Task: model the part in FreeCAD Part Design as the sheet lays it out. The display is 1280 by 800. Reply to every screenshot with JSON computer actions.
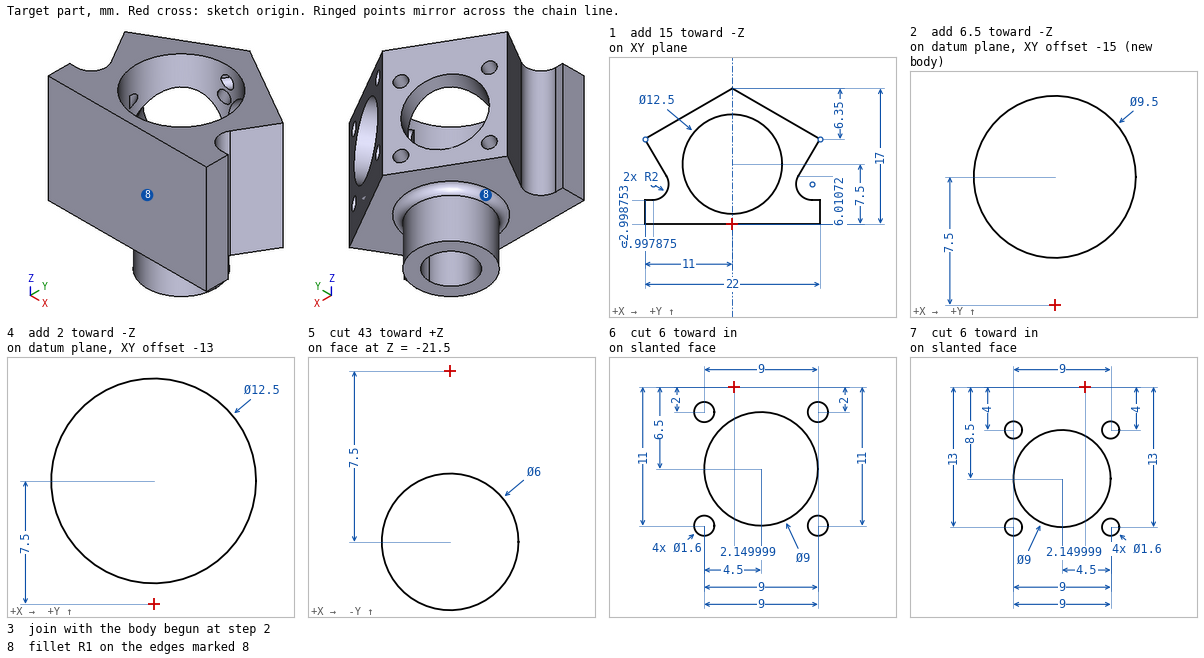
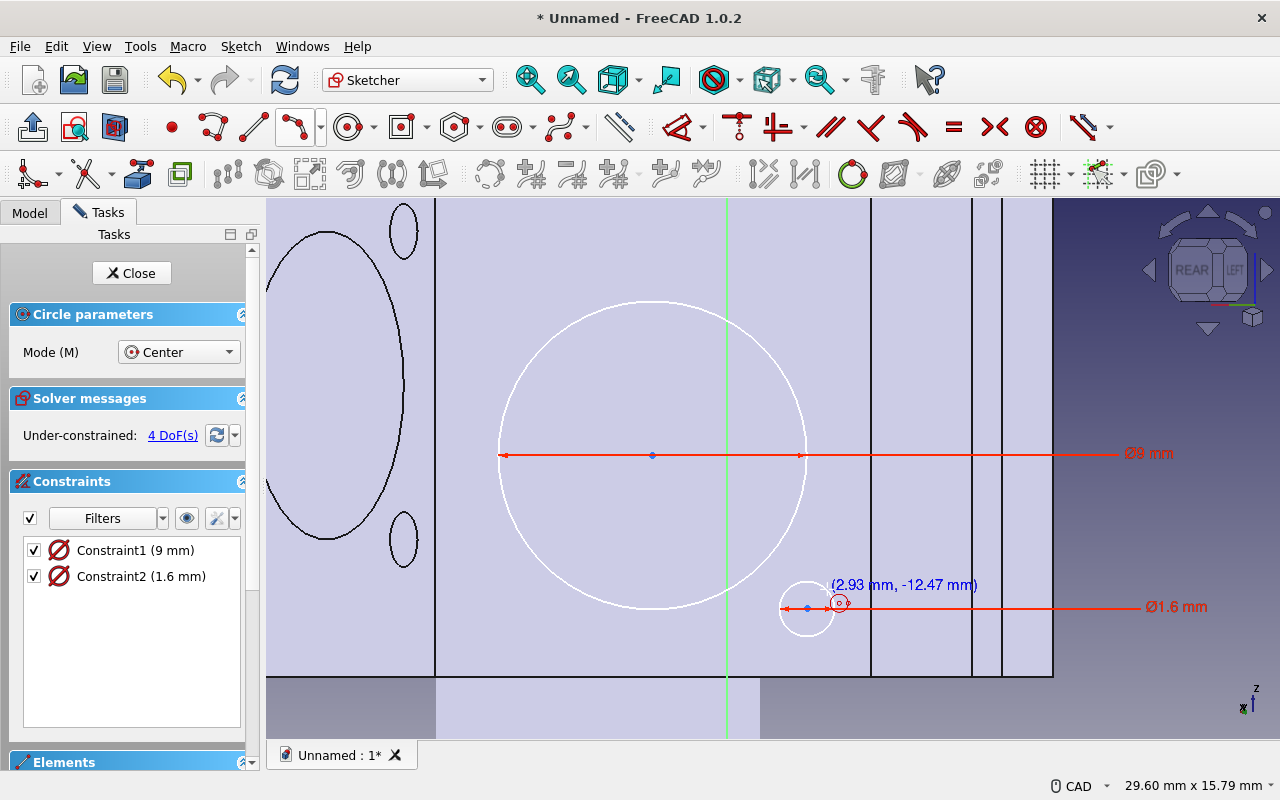
{"action": "left_click", "coordinate": [499, 608]}
{"action": "mouse_move", "coordinate": [518, 589]}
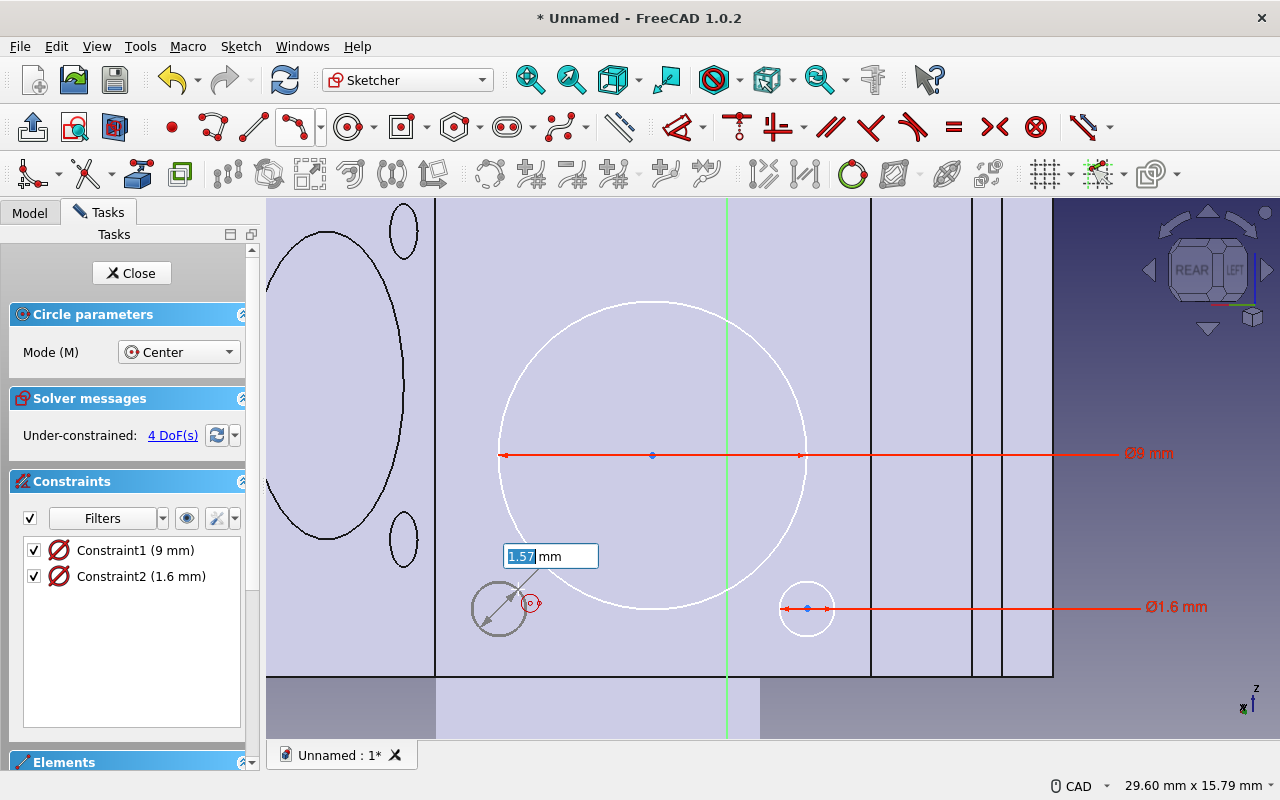
{"action": "type", "text": "1.6"}
{"action": "key", "text": "Return"}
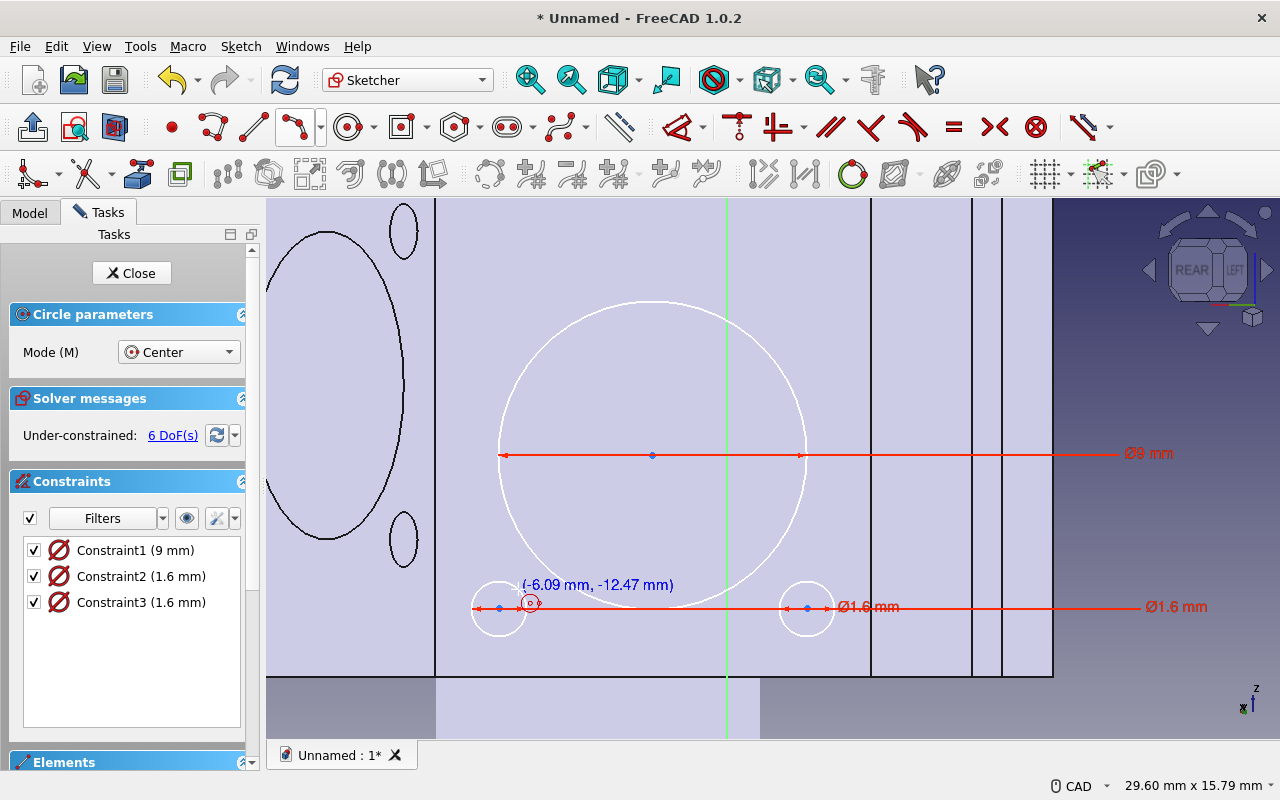
{"action": "left_click", "coordinate": [499, 300]}
{"action": "mouse_move", "coordinate": [518, 280]}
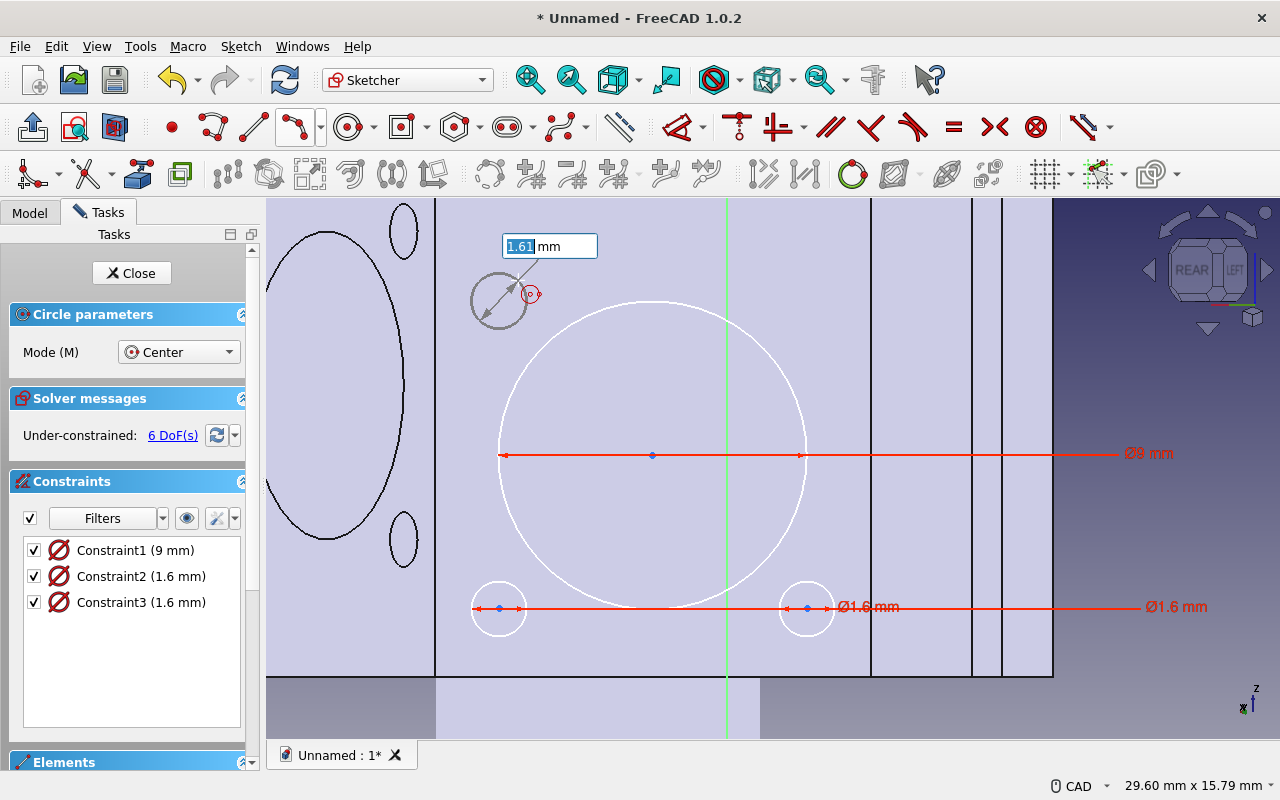
{"action": "type", "text": "1.6"}
{"action": "key", "text": "Return"}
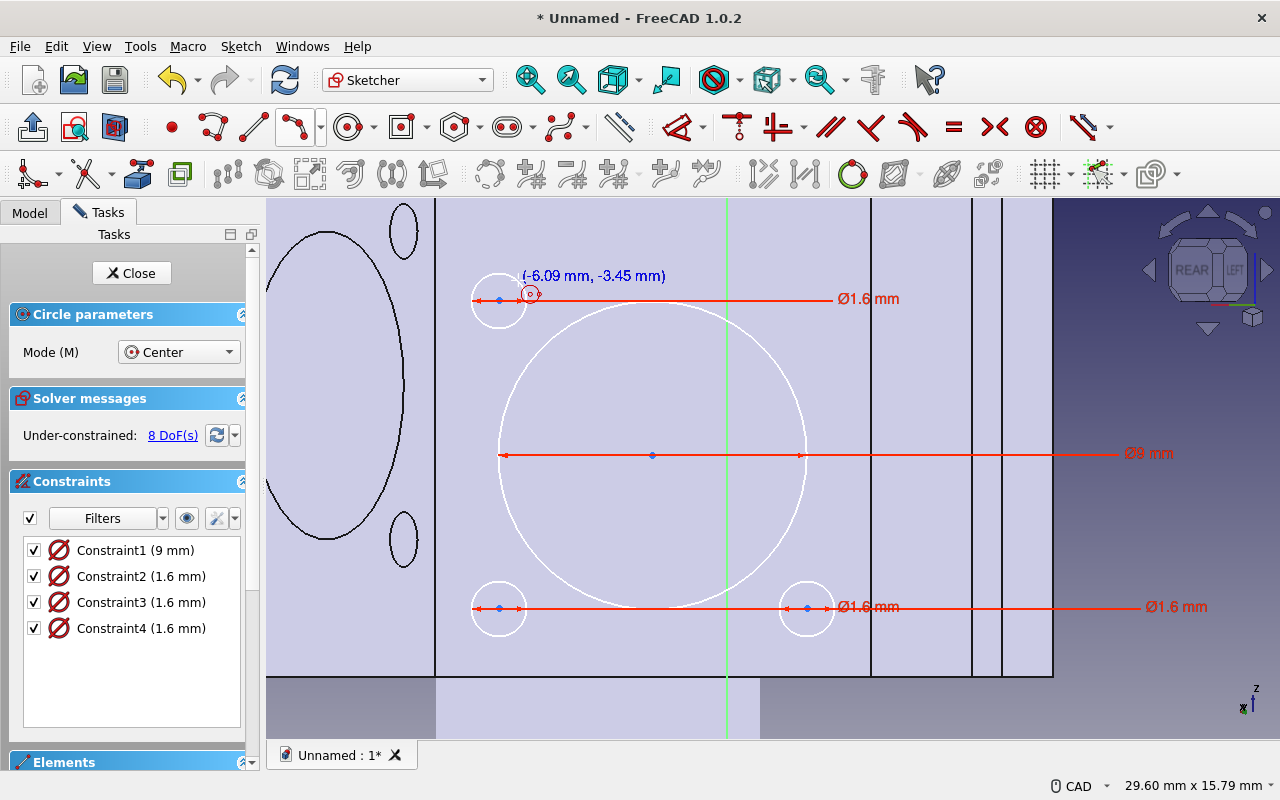
{"action": "left_click", "coordinate": [807, 300]}
{"action": "mouse_move", "coordinate": [827, 280]}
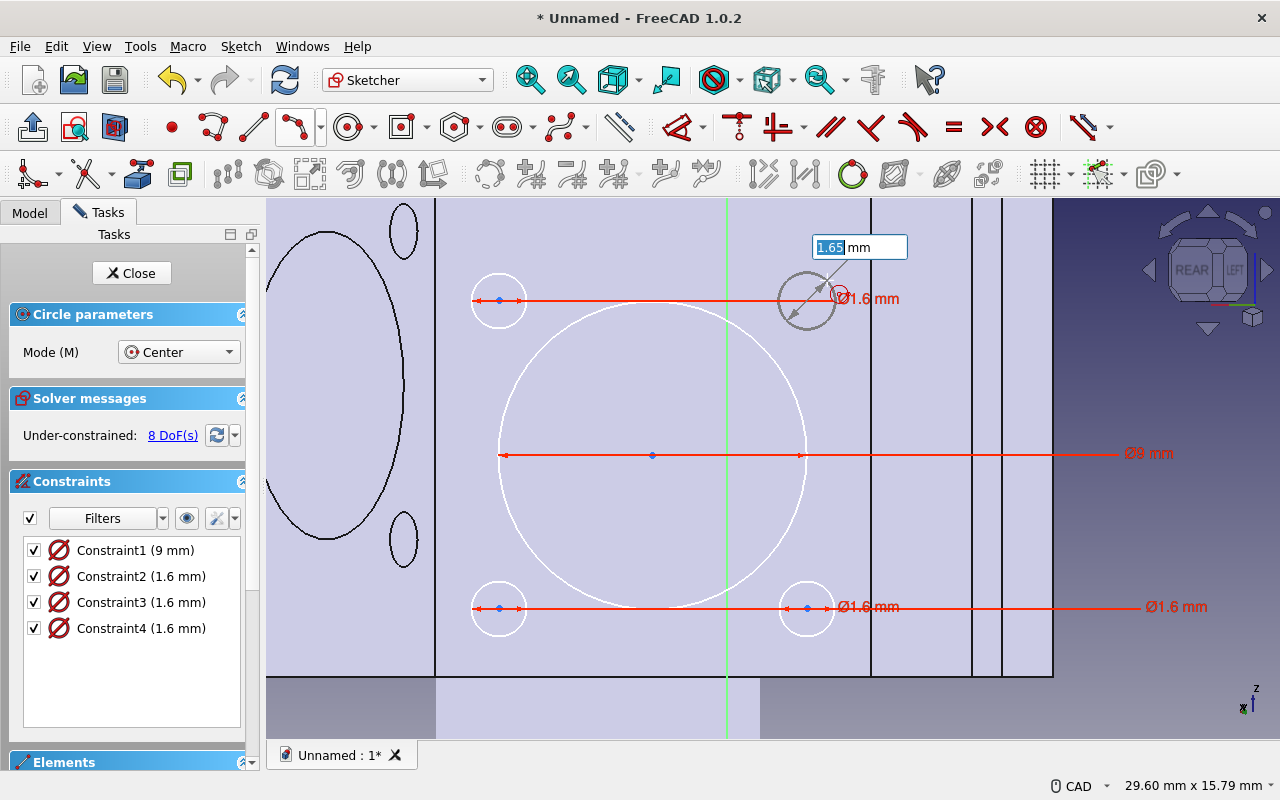
{"action": "type", "text": "1.6"}
{"action": "key", "text": "Return"}
{"action": "key", "text": "Escape"}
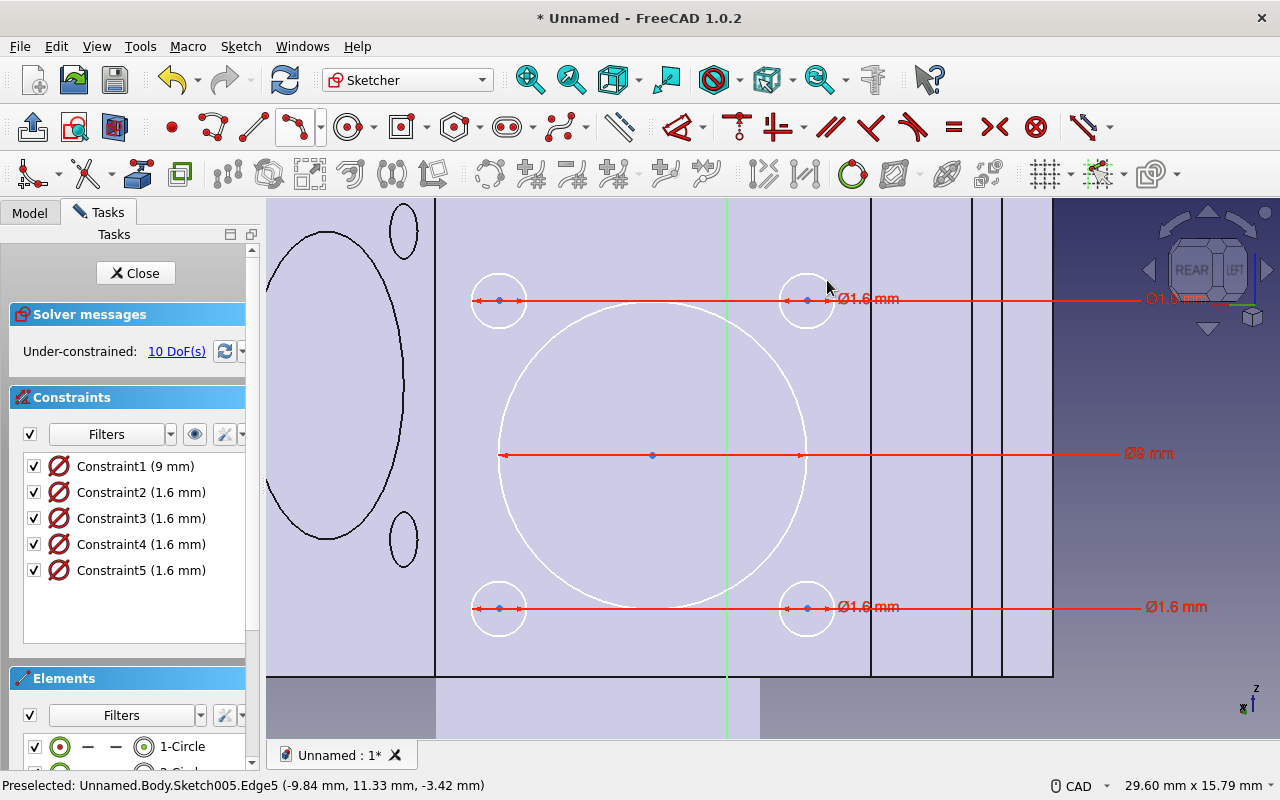
{"action": "left_click", "coordinate": [676, 128]}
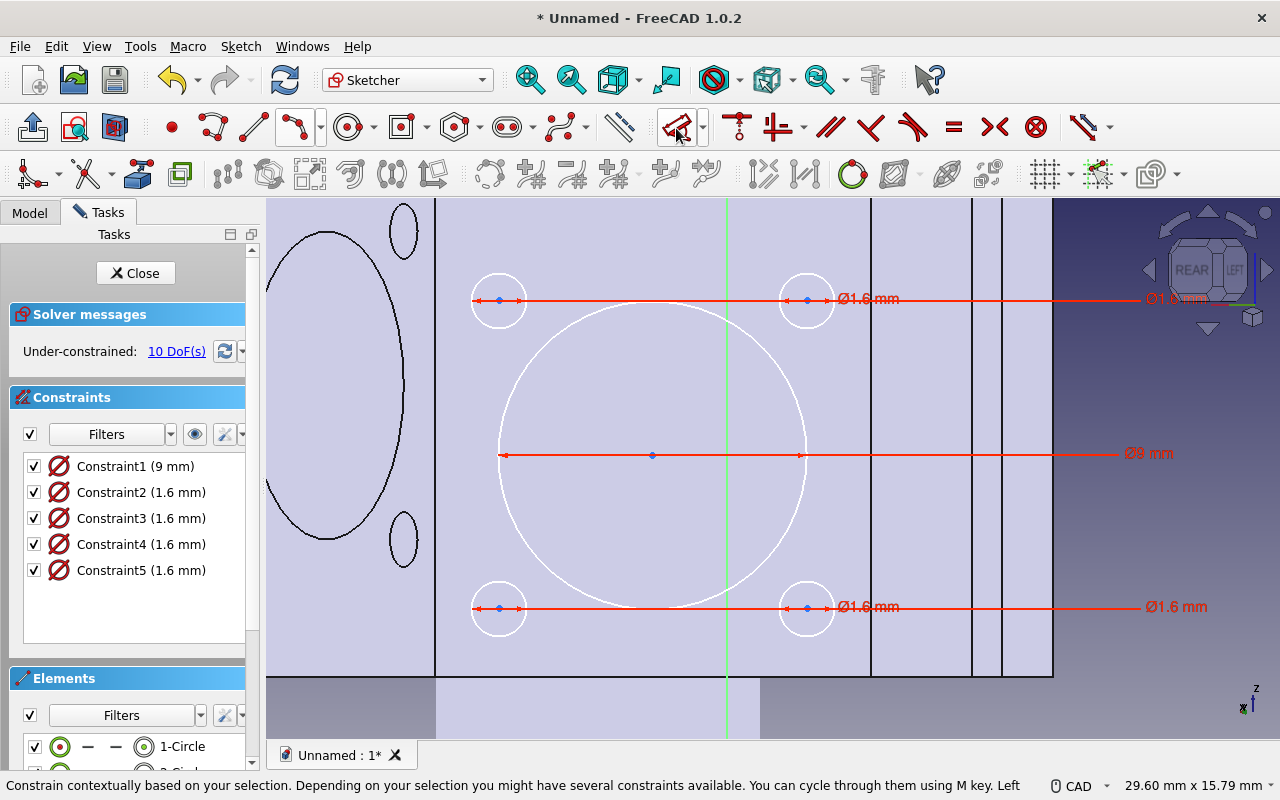
{"action": "left_click", "coordinate": [499, 301]}
{"action": "left_click", "coordinate": [465, 263]}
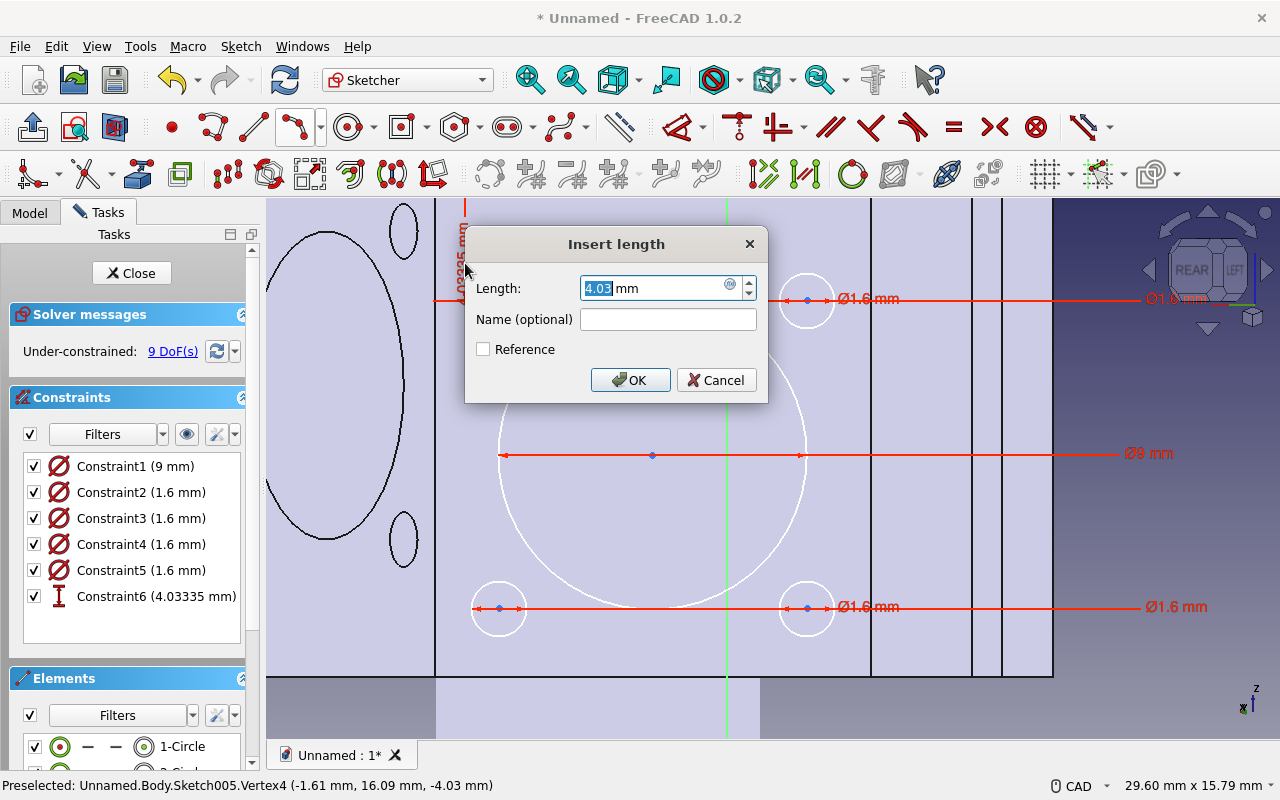
{"action": "type", "text": "4"}
{"action": "key", "text": "Return"}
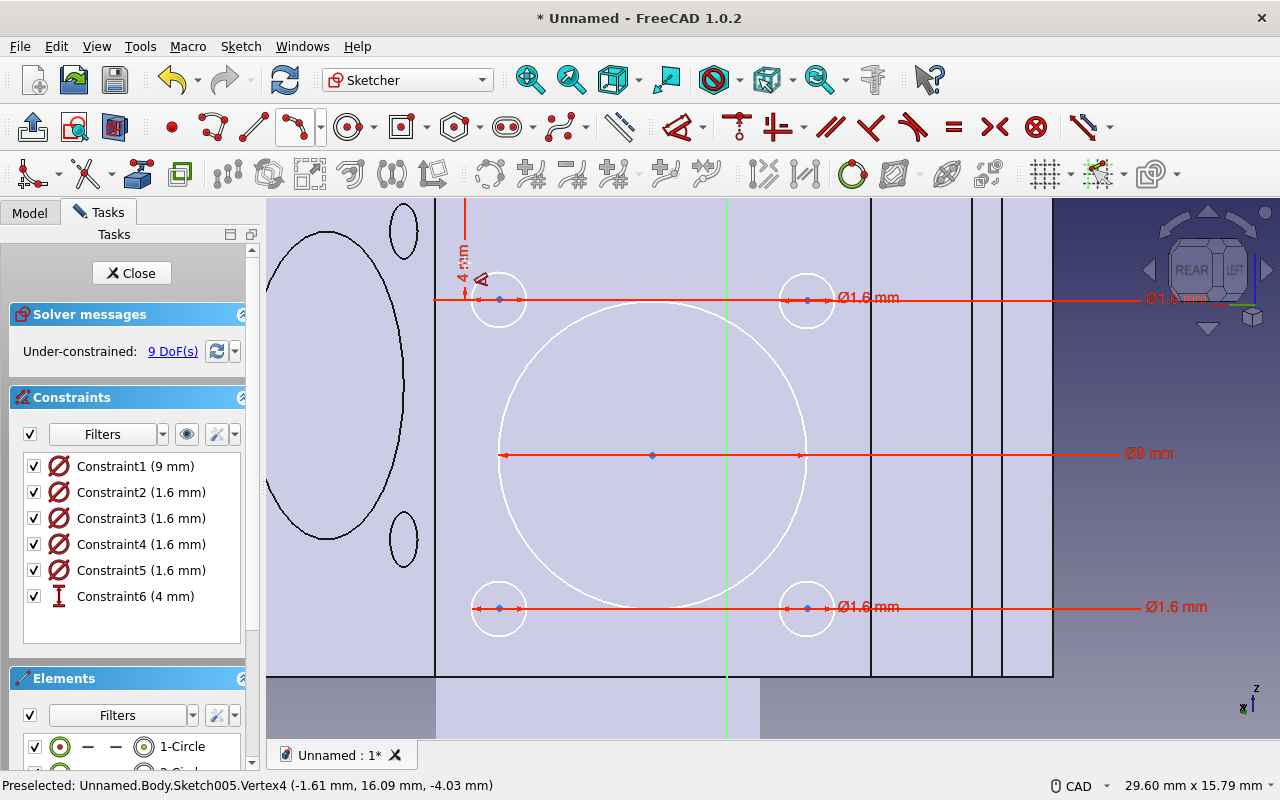
{"action": "left_click", "coordinate": [807, 301]}
{"action": "left_click", "coordinate": [841, 263]}